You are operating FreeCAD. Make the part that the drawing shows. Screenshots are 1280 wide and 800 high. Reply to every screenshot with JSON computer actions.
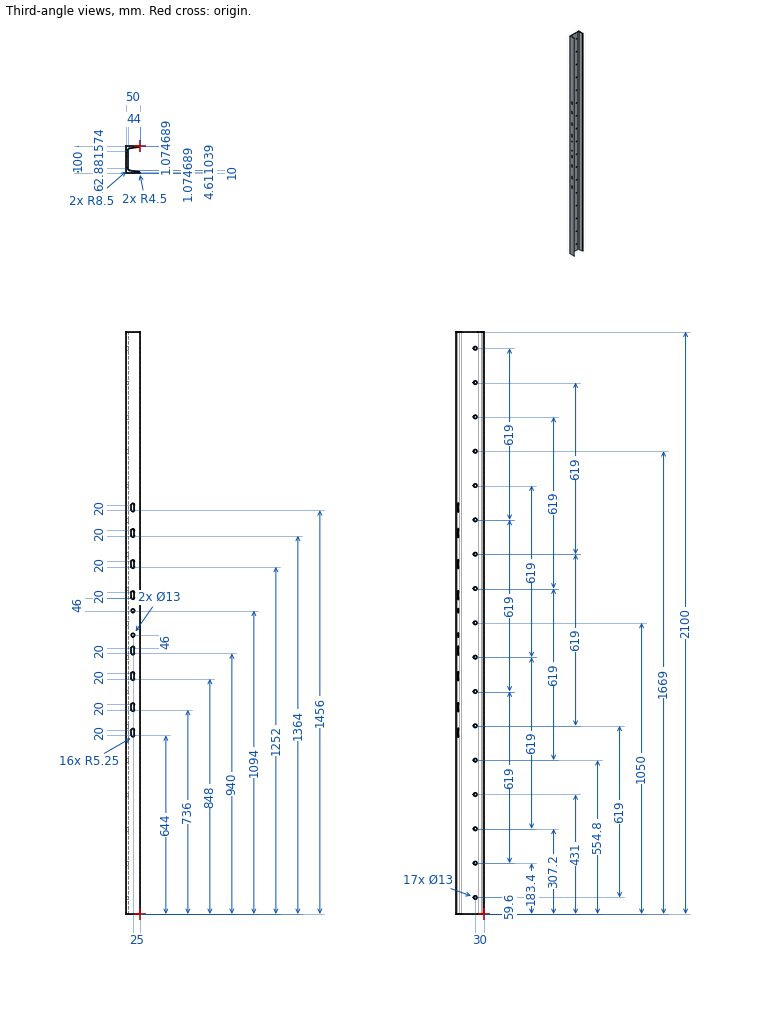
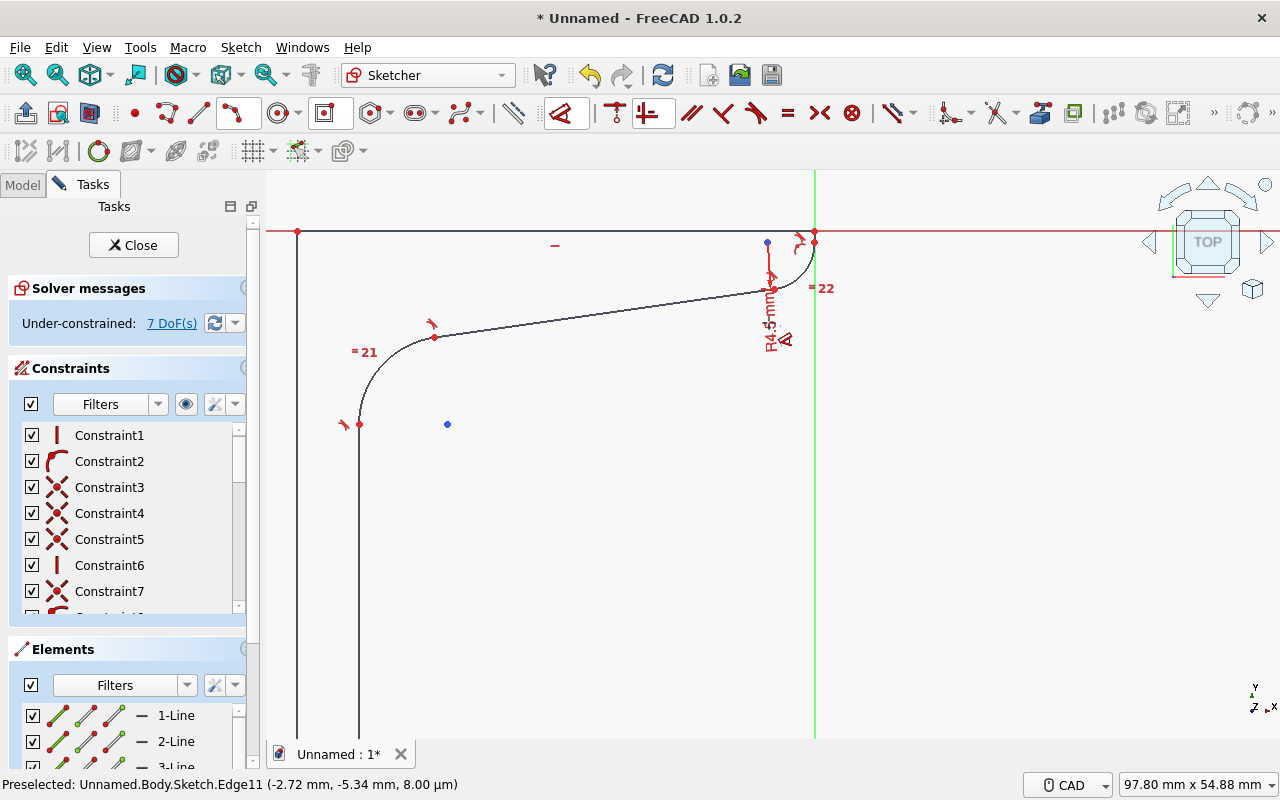
{"action": "left_click", "coordinate": [659, 231]}
{"action": "left_click", "coordinate": [556, 265]}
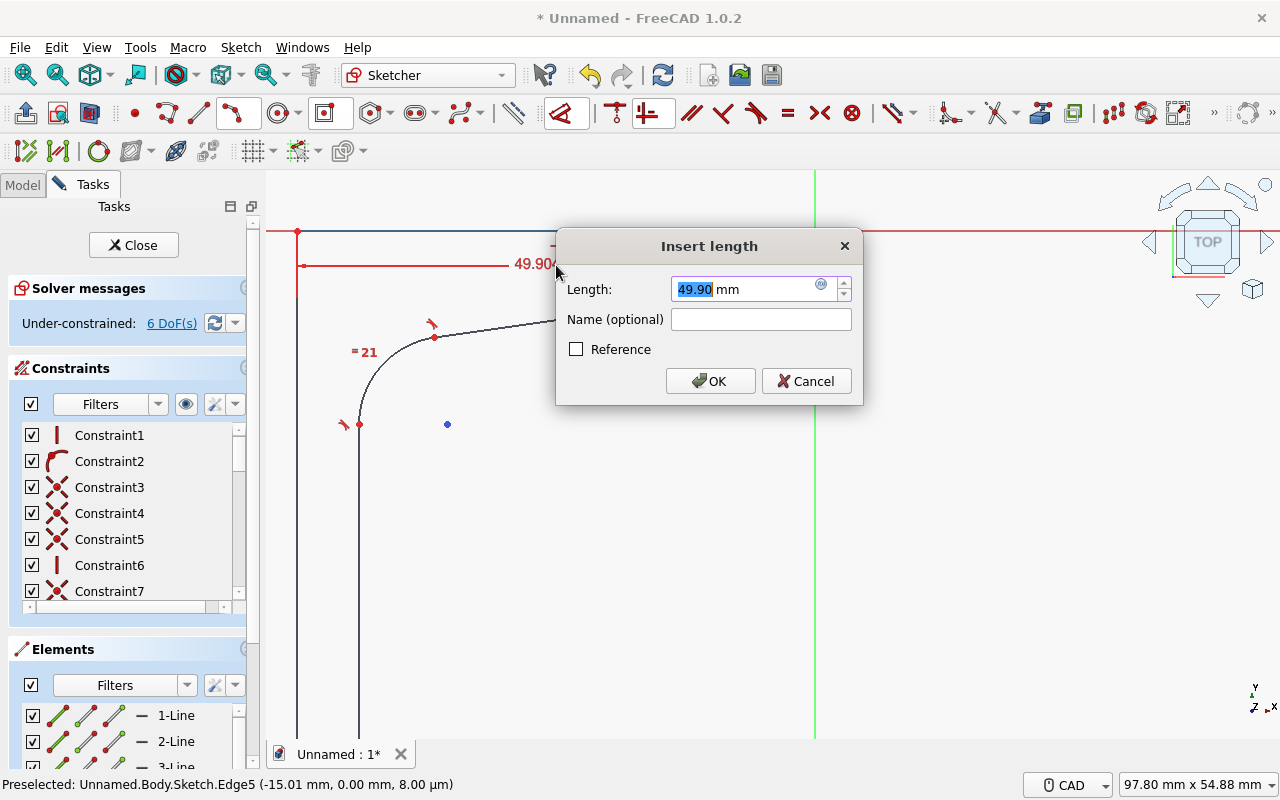
{"action": "type", "text": "50"}
{"action": "key", "text": "Return"}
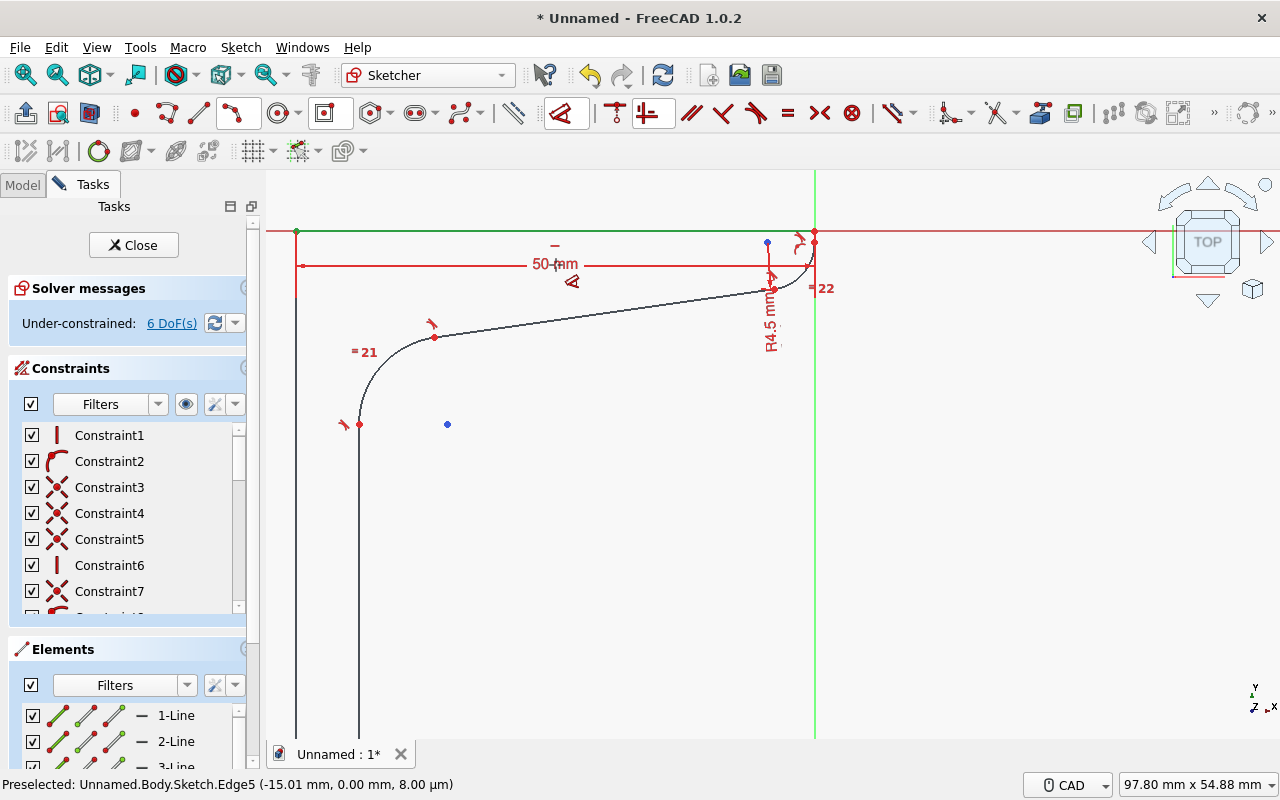
{"action": "left_click", "coordinate": [296, 544]}
{"action": "left_click", "coordinate": [330, 471]}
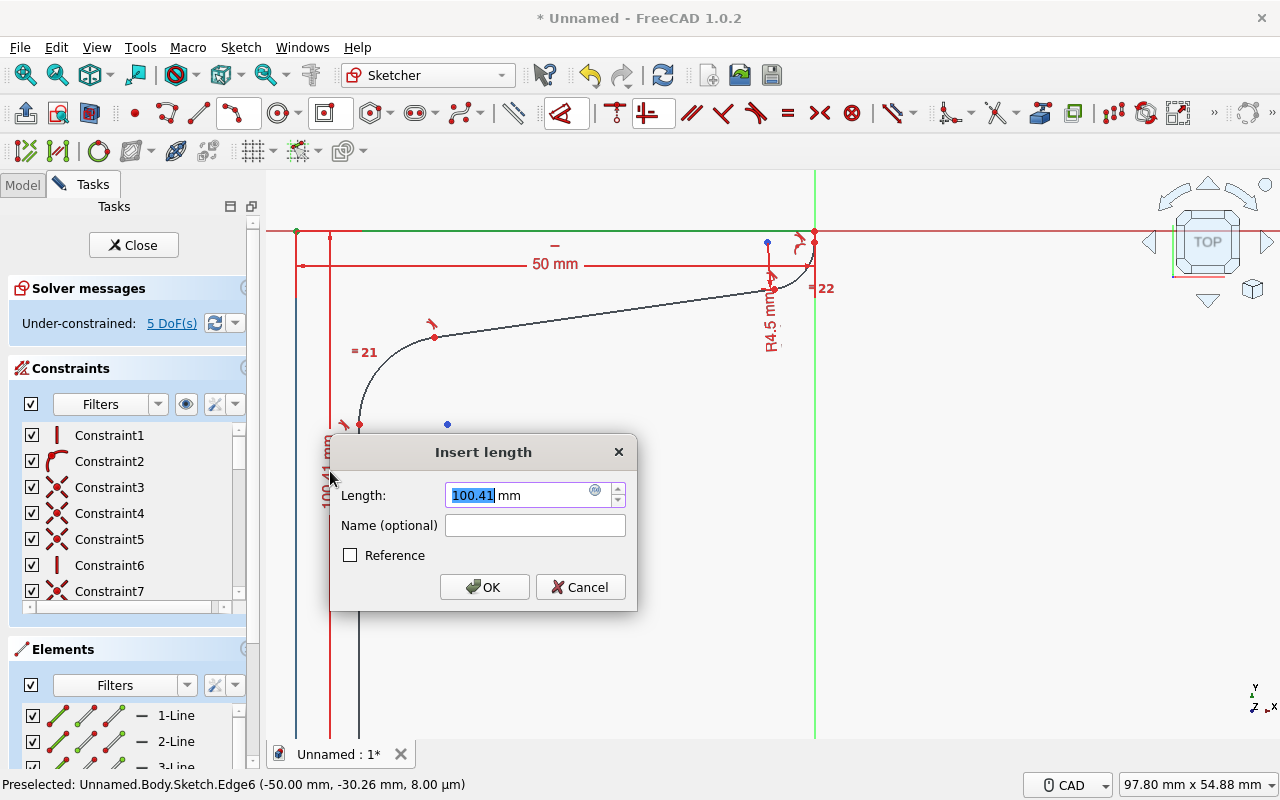
{"action": "type", "text": "100"}
{"action": "key", "text": "Return"}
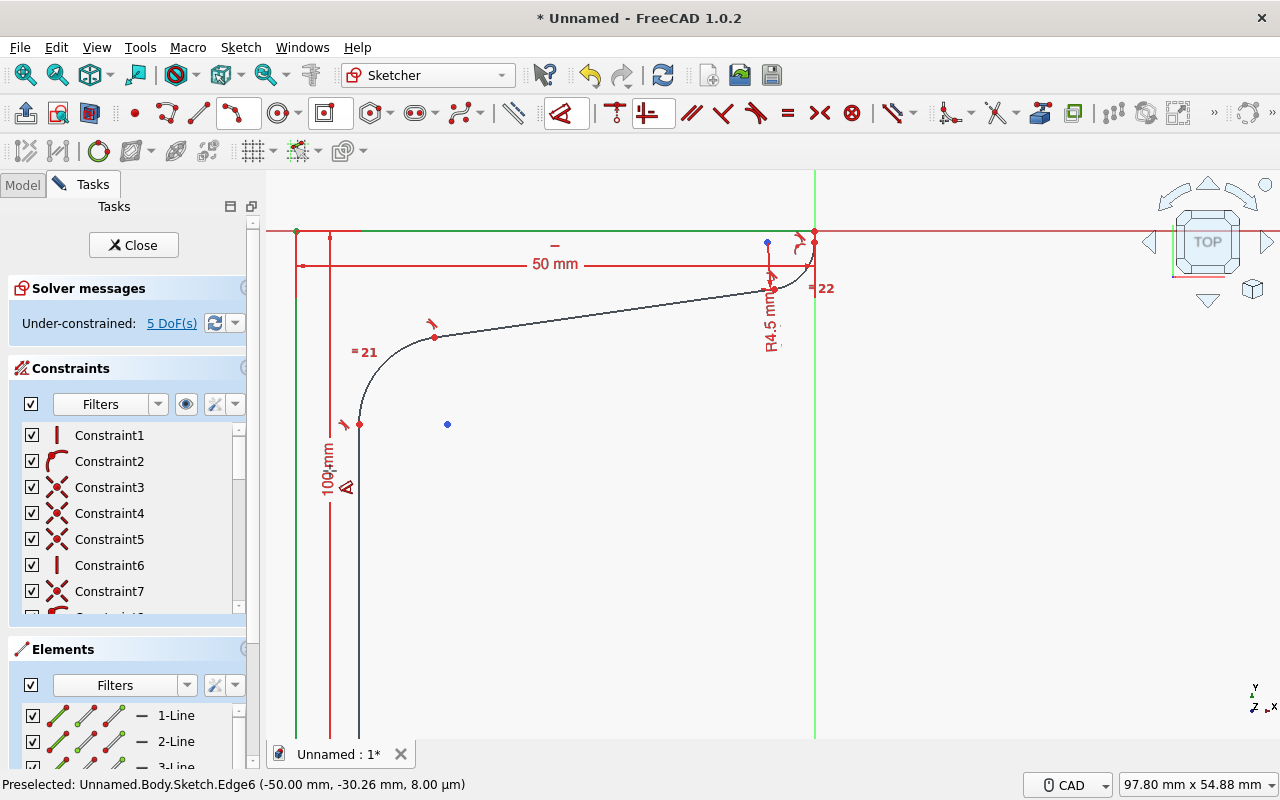
{"action": "scroll", "coordinate": [791, 283], "scroll_direction": "down", "scroll_amount": 5}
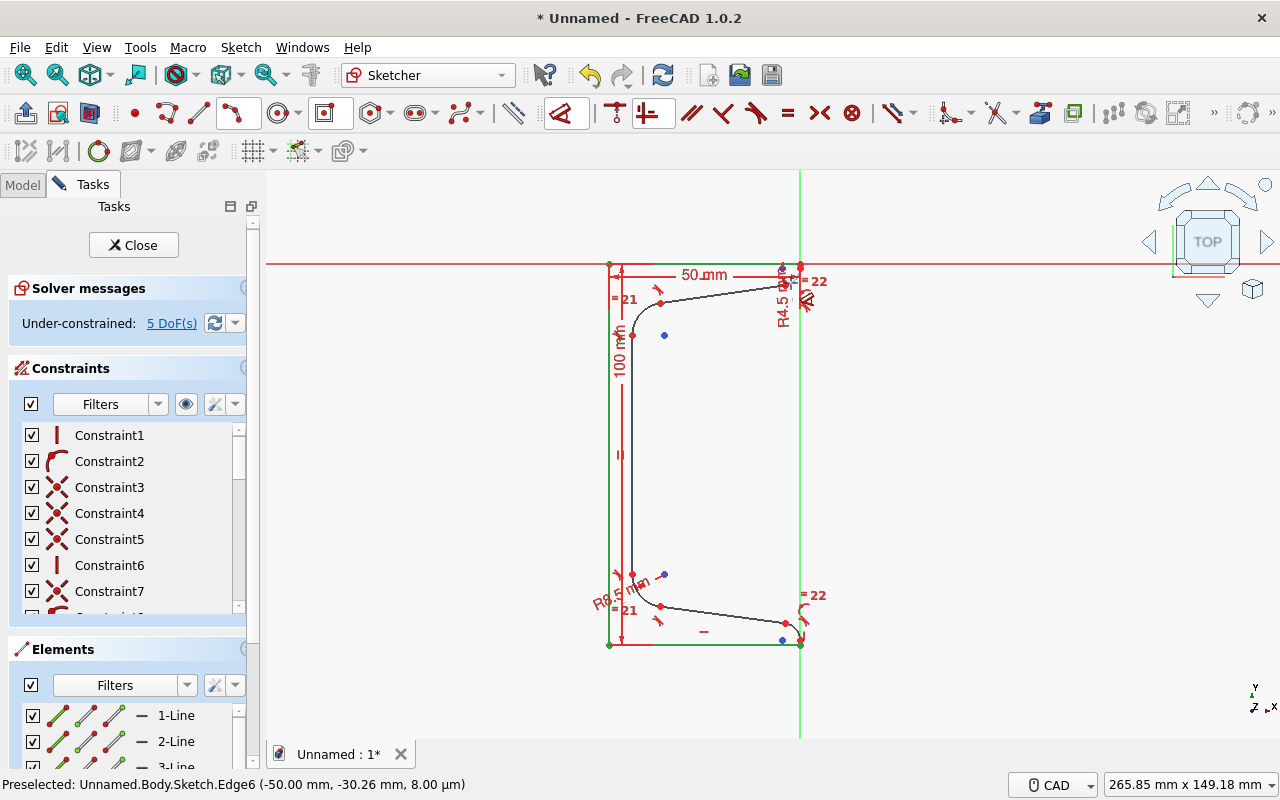
{"action": "left_click", "coordinate": [632, 575]}
{"action": "left_click", "coordinate": [716, 230]}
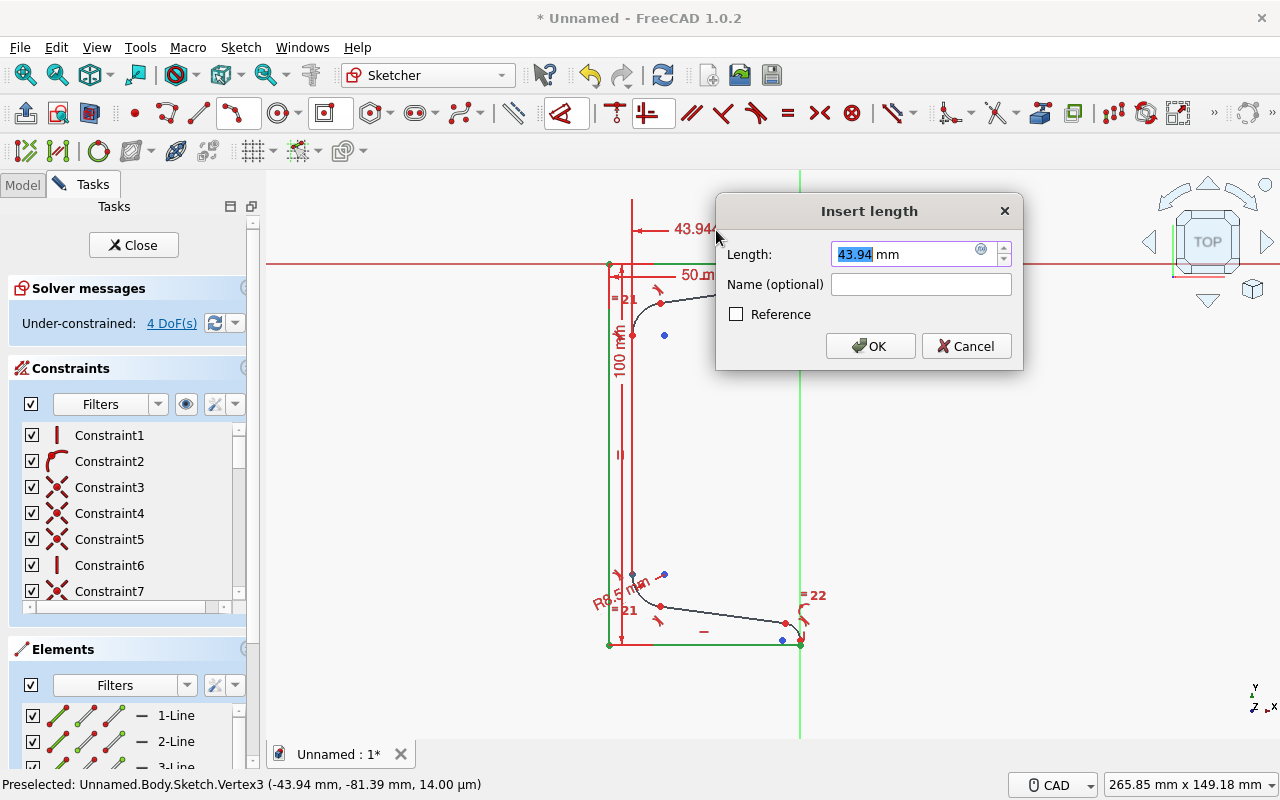
{"action": "type", "text": "44"}
{"action": "key", "text": "Return"}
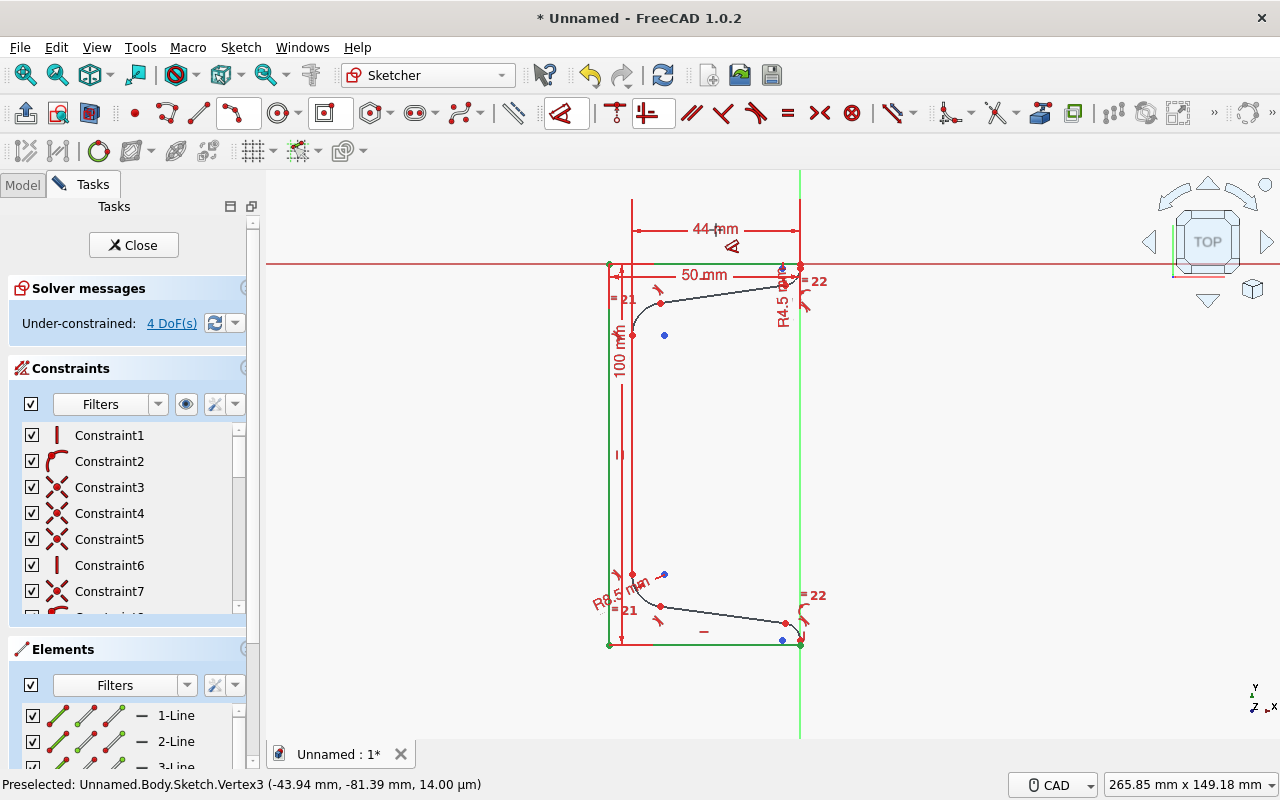
{"action": "scroll", "coordinate": [800, 266], "scroll_direction": "up", "scroll_amount": 12}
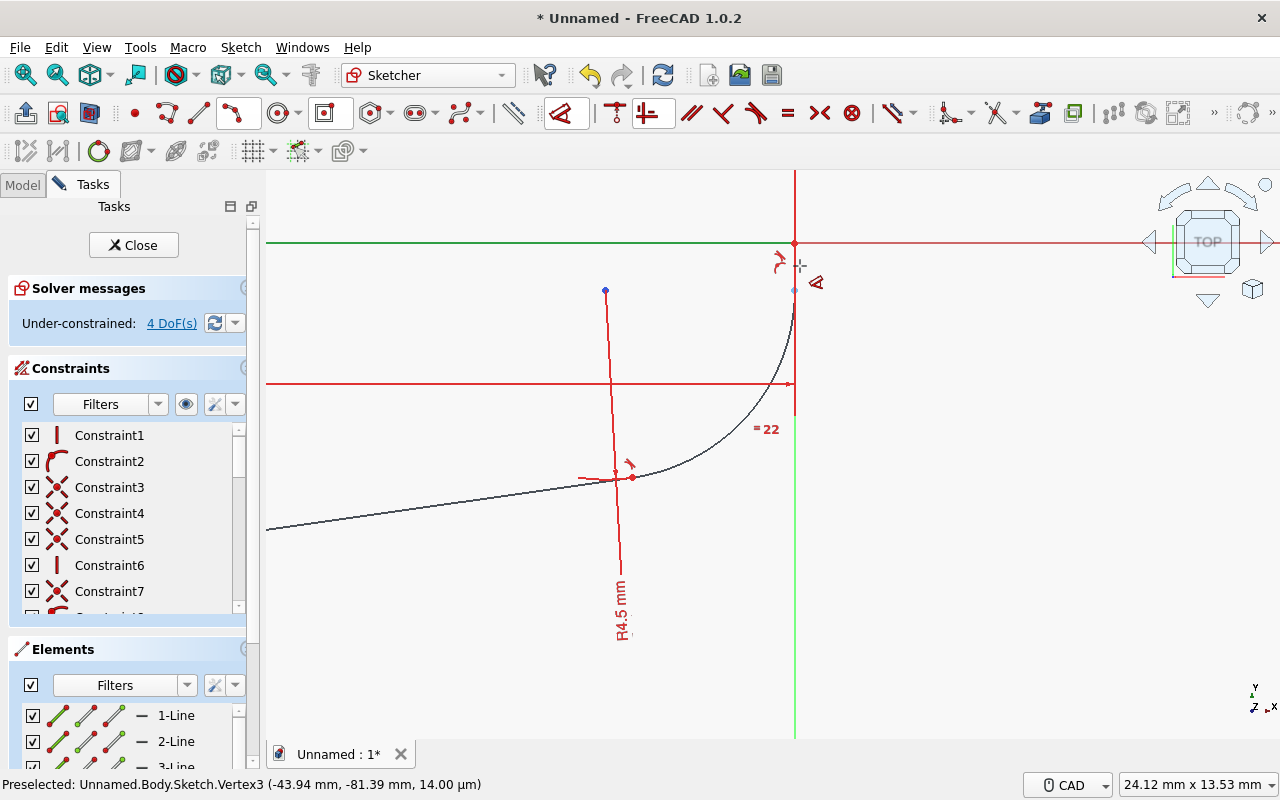
{"action": "left_click", "coordinate": [795, 267]}
{"action": "left_click", "coordinate": [829, 267]}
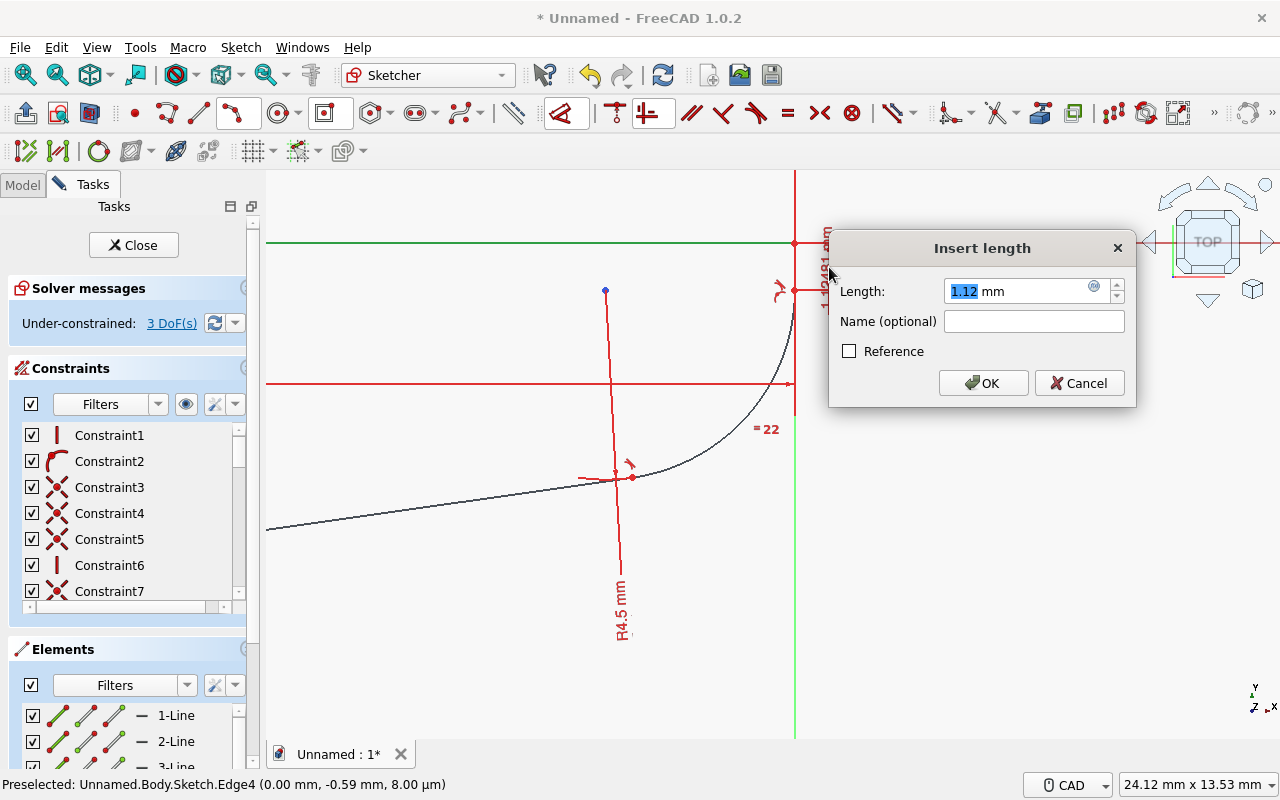
{"action": "type", "text": "1.074689"}
{"action": "key", "text": "Return"}